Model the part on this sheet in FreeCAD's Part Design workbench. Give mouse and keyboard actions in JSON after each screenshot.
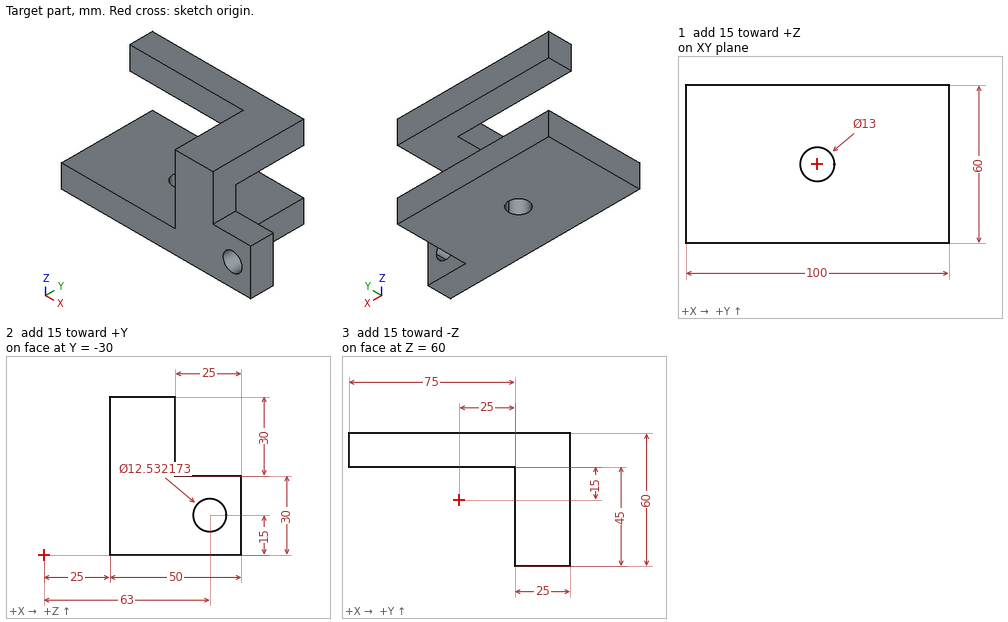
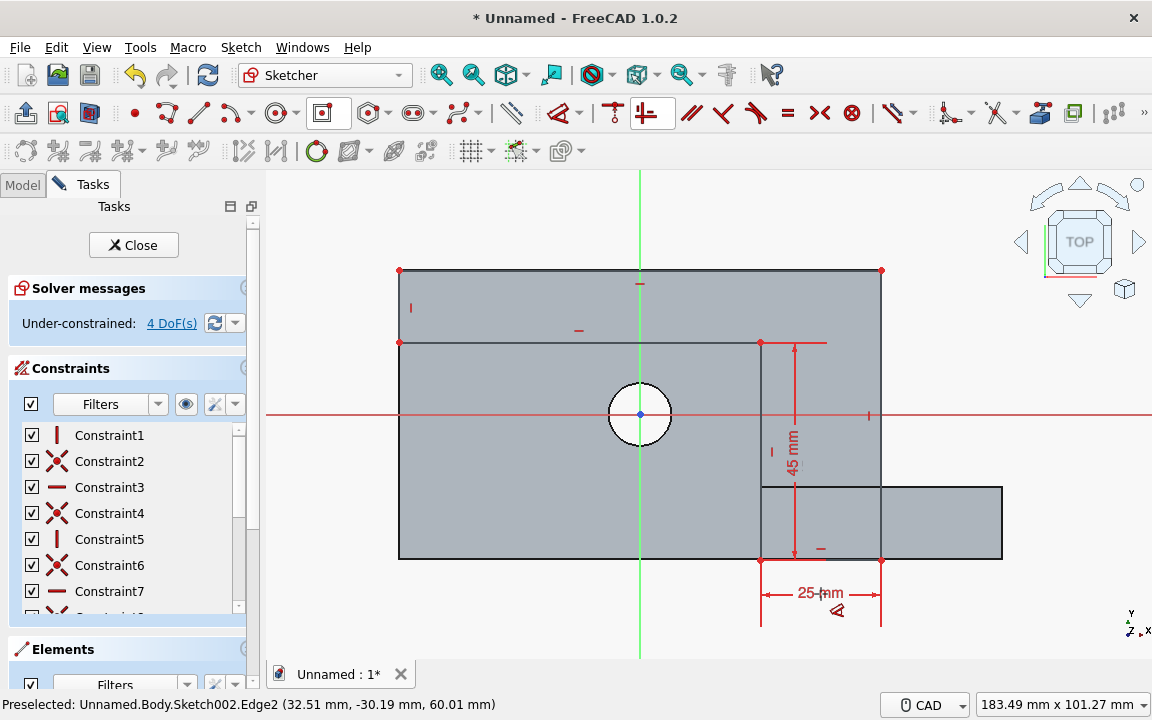
{"action": "left_click", "coordinate": [881, 474]}
{"action": "left_click", "coordinate": [915, 349]}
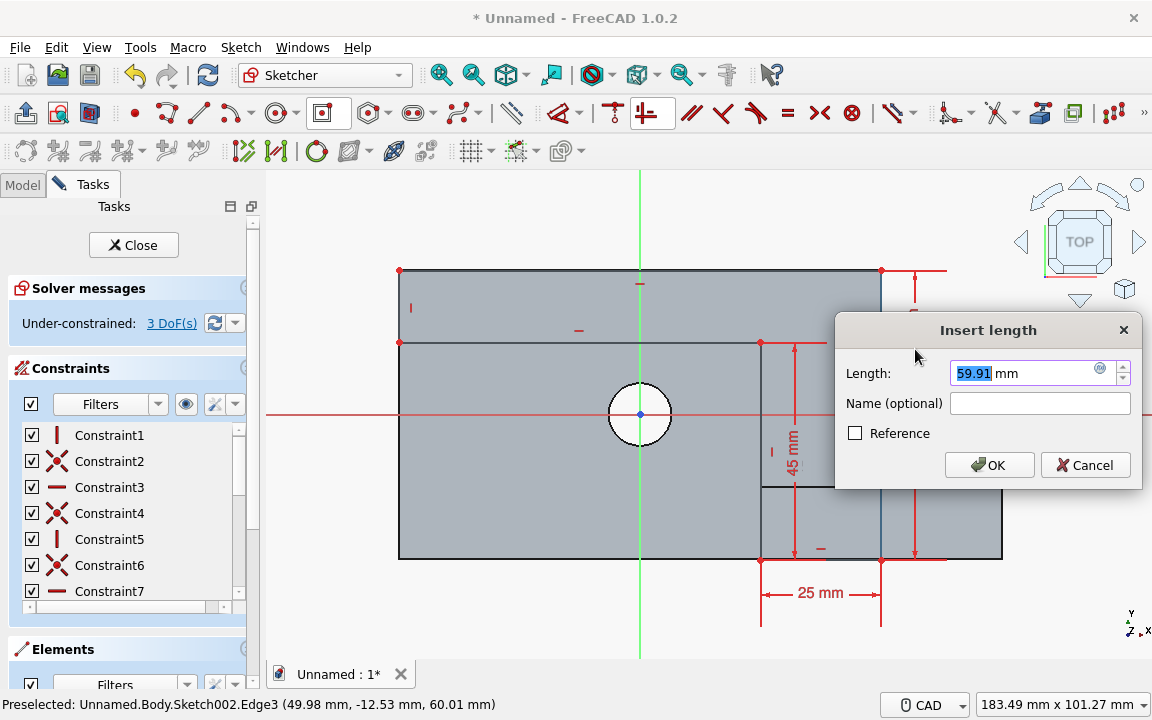
{"action": "type", "text": "60"}
{"action": "key", "text": "Return"}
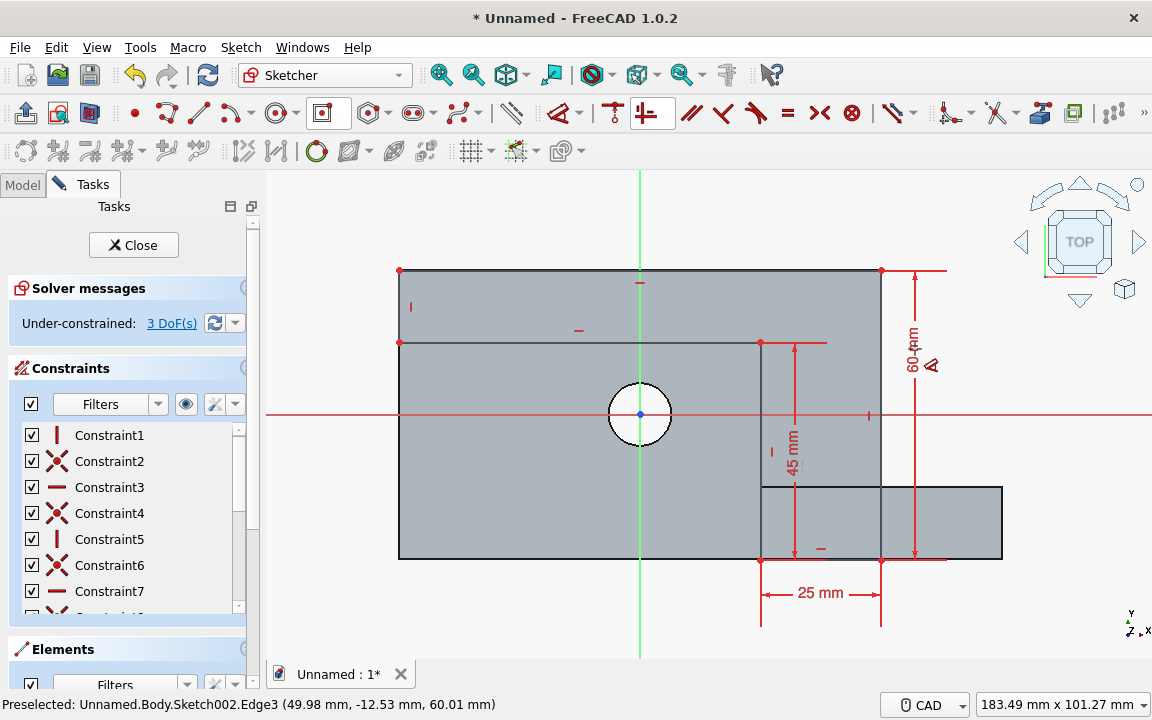
{"action": "left_click", "coordinate": [507, 343]}
{"action": "left_click", "coordinate": [580, 309]}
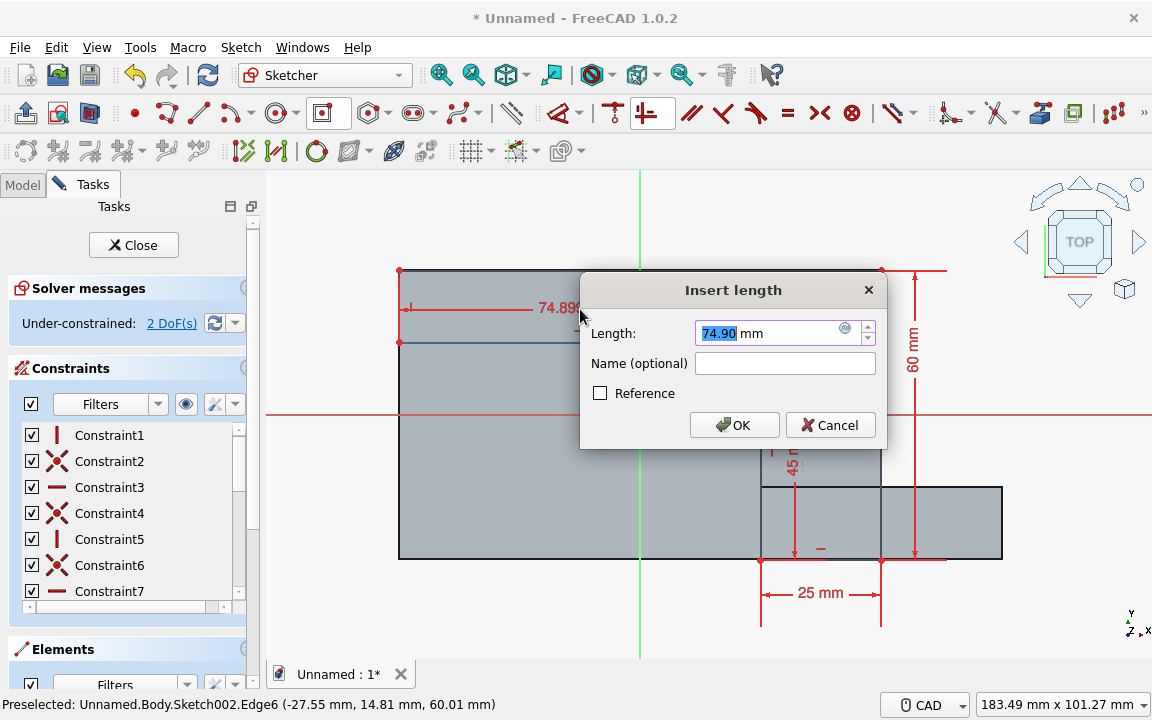
{"action": "type", "text": "75"}
{"action": "key", "text": "Return"}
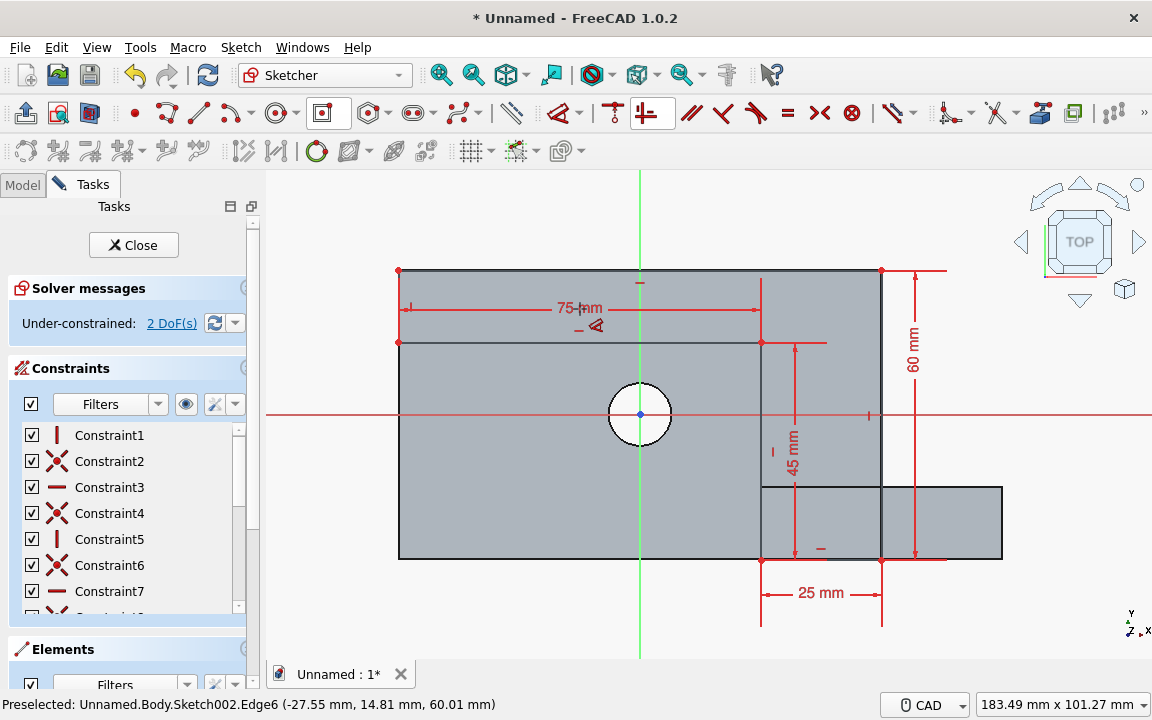
{"action": "left_click", "coordinate": [761, 343]}
{"action": "left_click", "coordinate": [701, 309]}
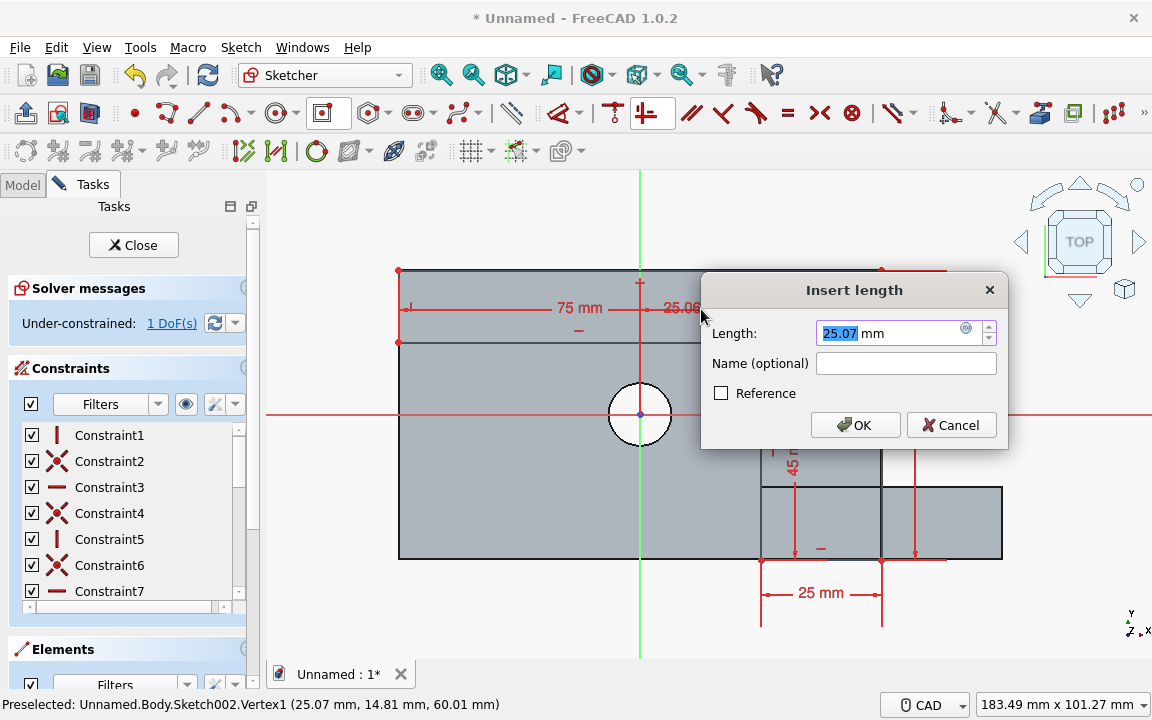
{"action": "type", "text": "25"}
{"action": "key", "text": "Return"}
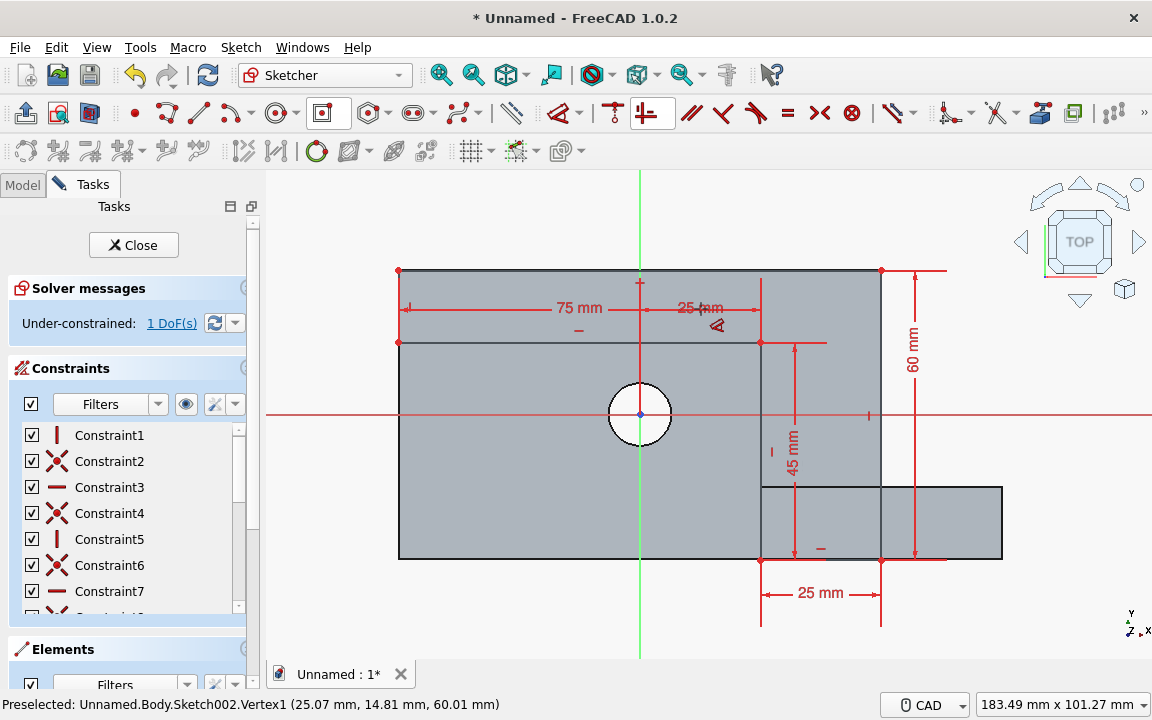
{"action": "left_click", "coordinate": [761, 343]}
{"action": "left_click", "coordinate": [795, 379]}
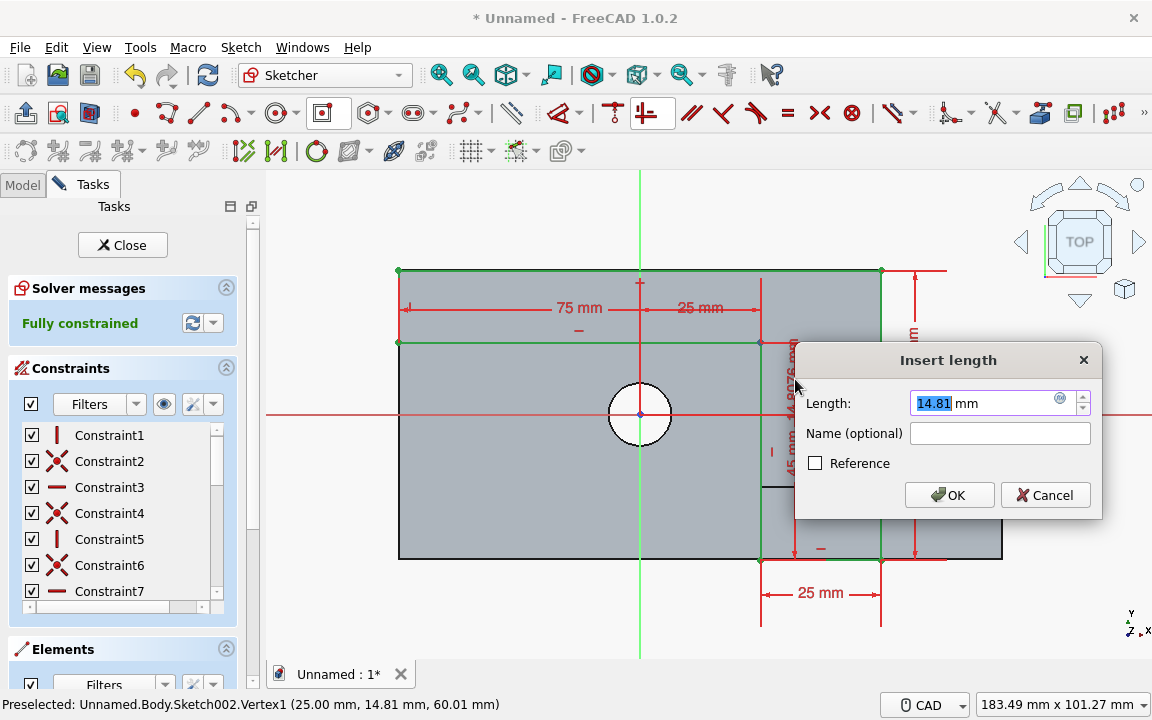
{"action": "type", "text": "15"}
{"action": "key", "text": "Return"}
{"action": "key", "text": "Escape"}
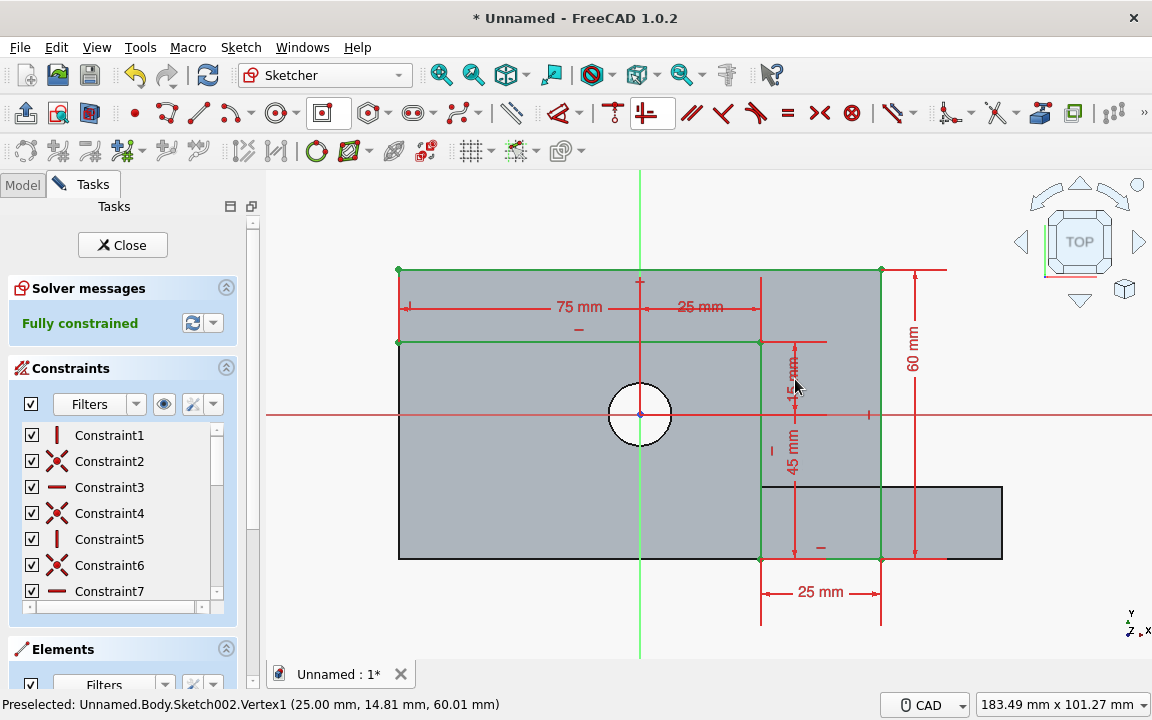
{"action": "left_click", "coordinate": [123, 245]}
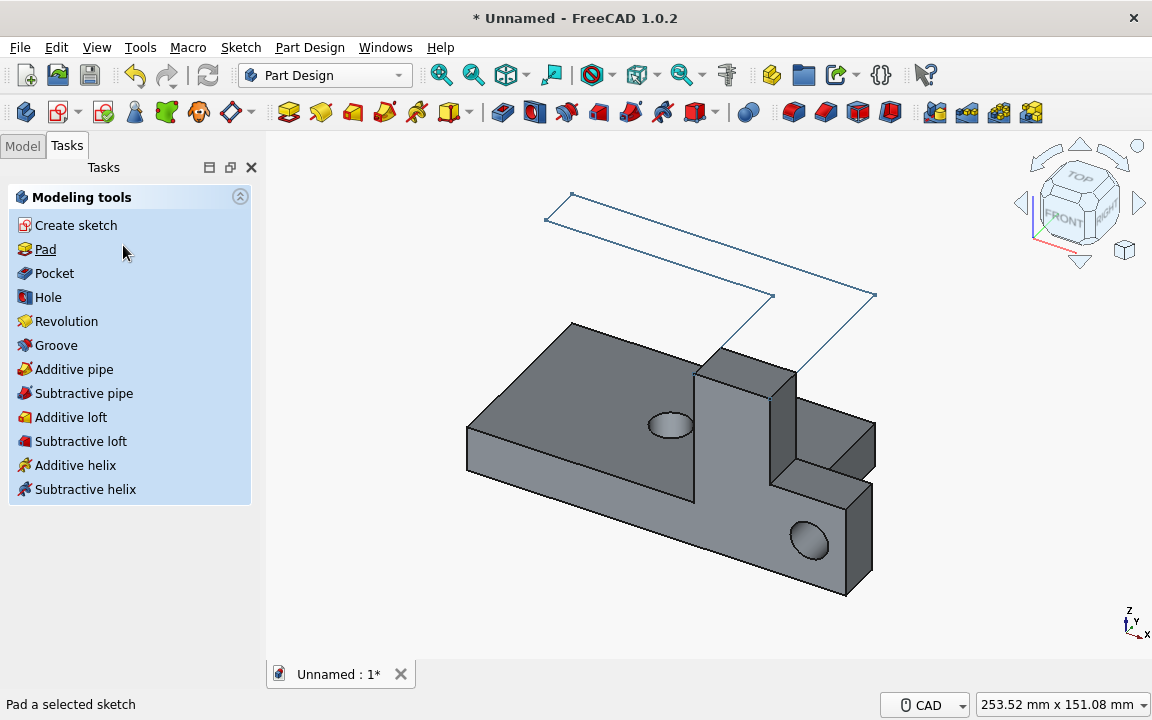
{"action": "left_click", "coordinate": [290, 112]}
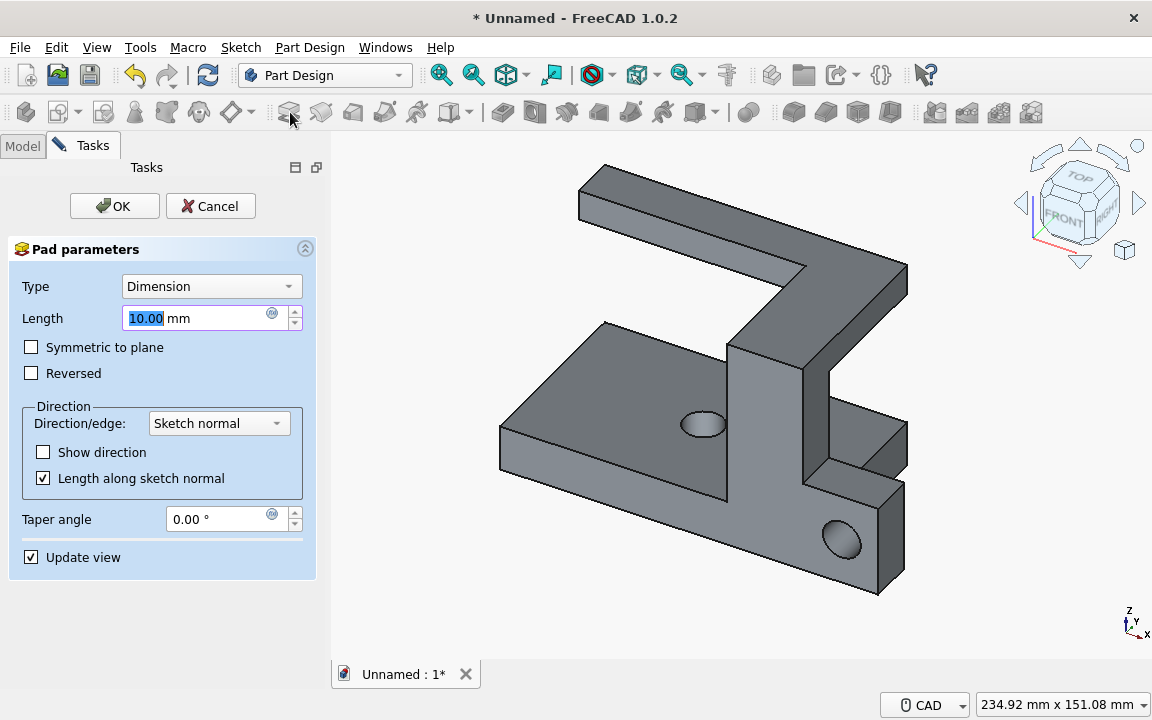
{"action": "type", "text": "15"}
{"action": "key", "text": "Tab"}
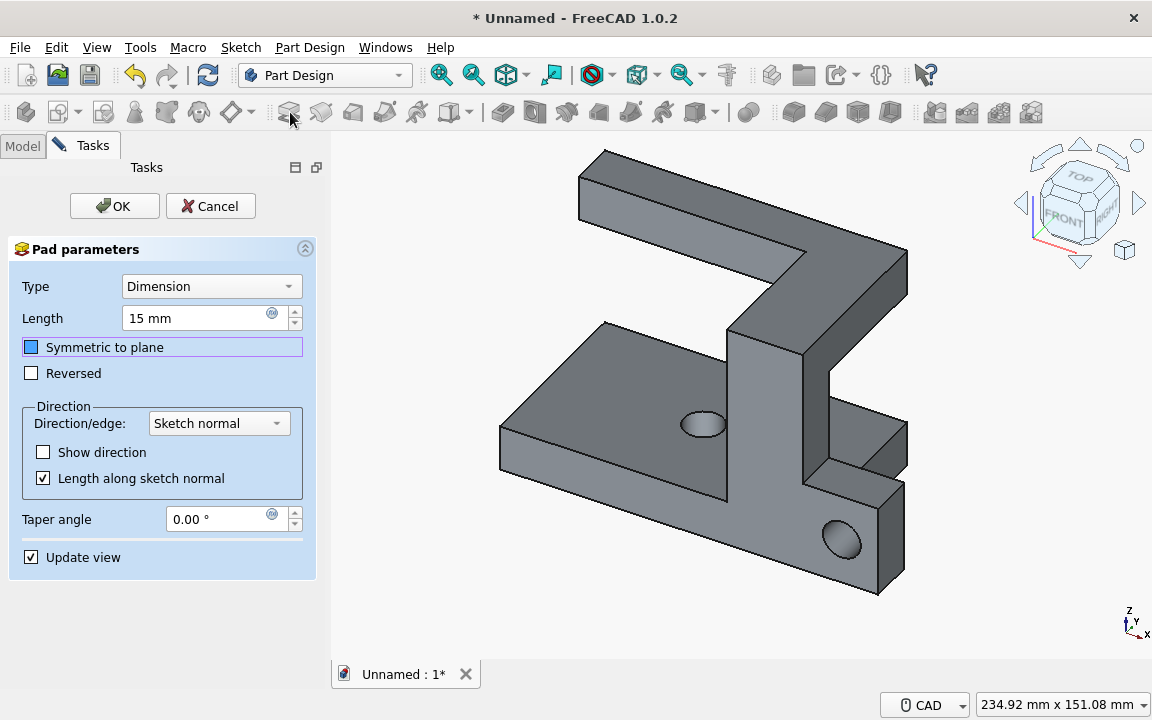
{"action": "left_click", "coordinate": [30, 373]}